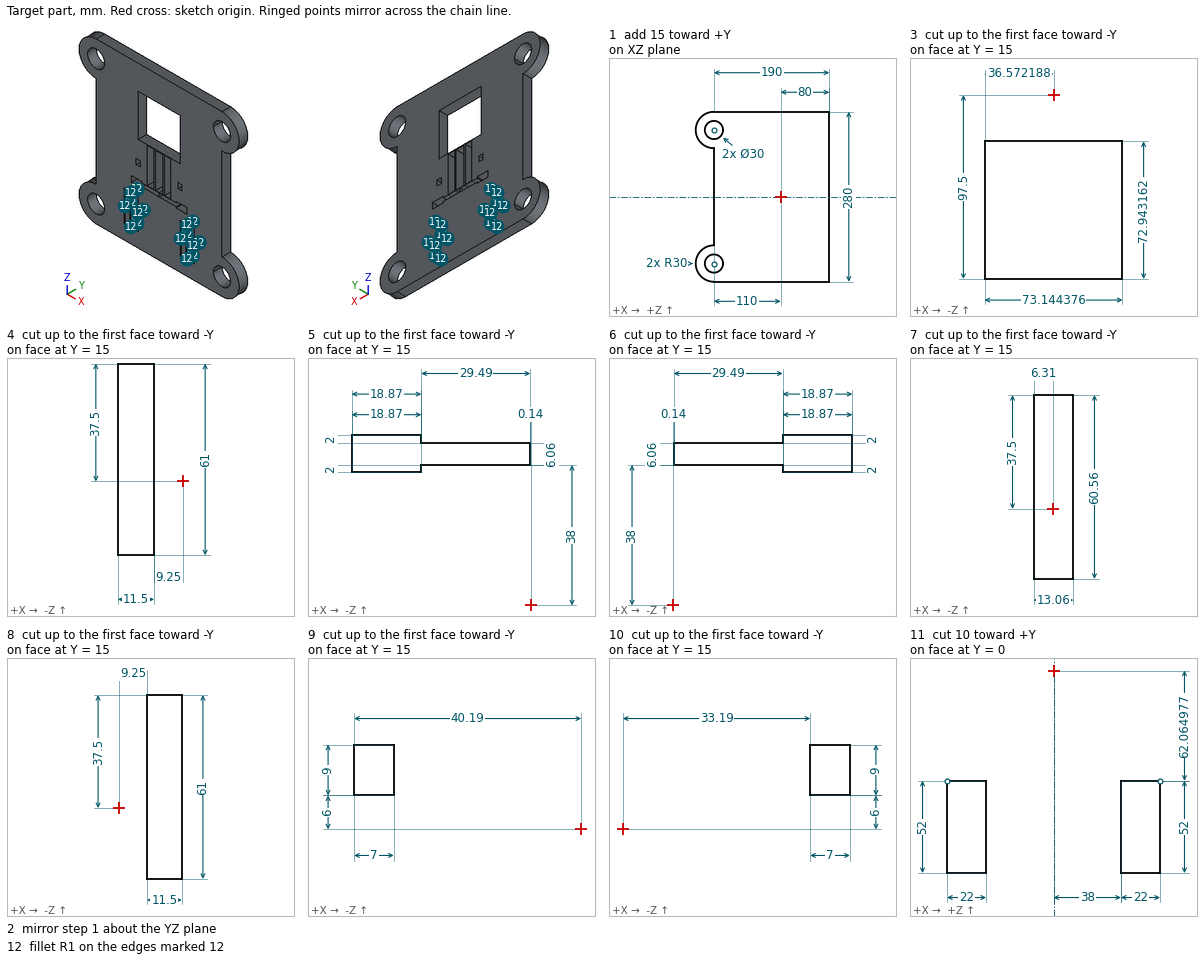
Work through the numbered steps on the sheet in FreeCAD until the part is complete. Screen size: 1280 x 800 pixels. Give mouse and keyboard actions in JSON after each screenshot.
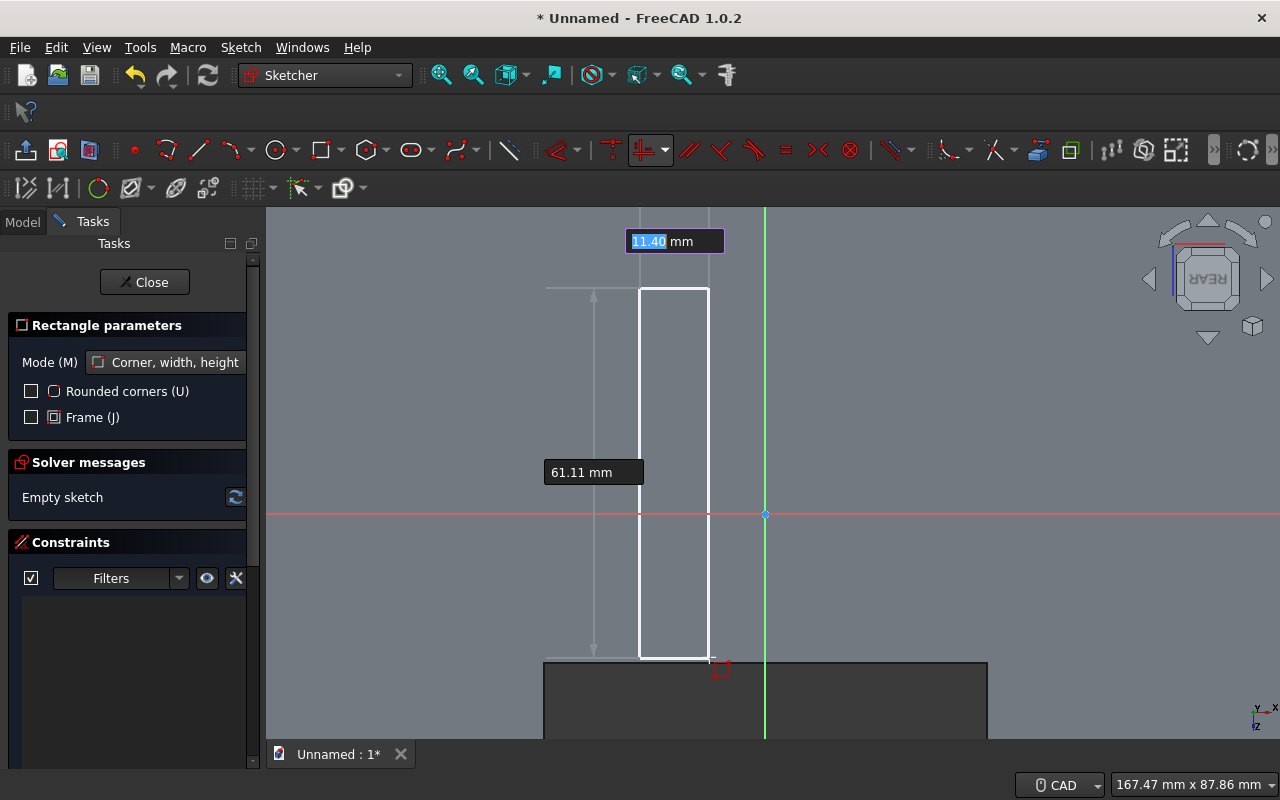
{"action": "type", "text": "11.5"}
{"action": "key", "text": "Tab"}
{"action": "type", "text": "61"}
{"action": "key", "text": "Return"}
{"action": "key", "text": "Escape"}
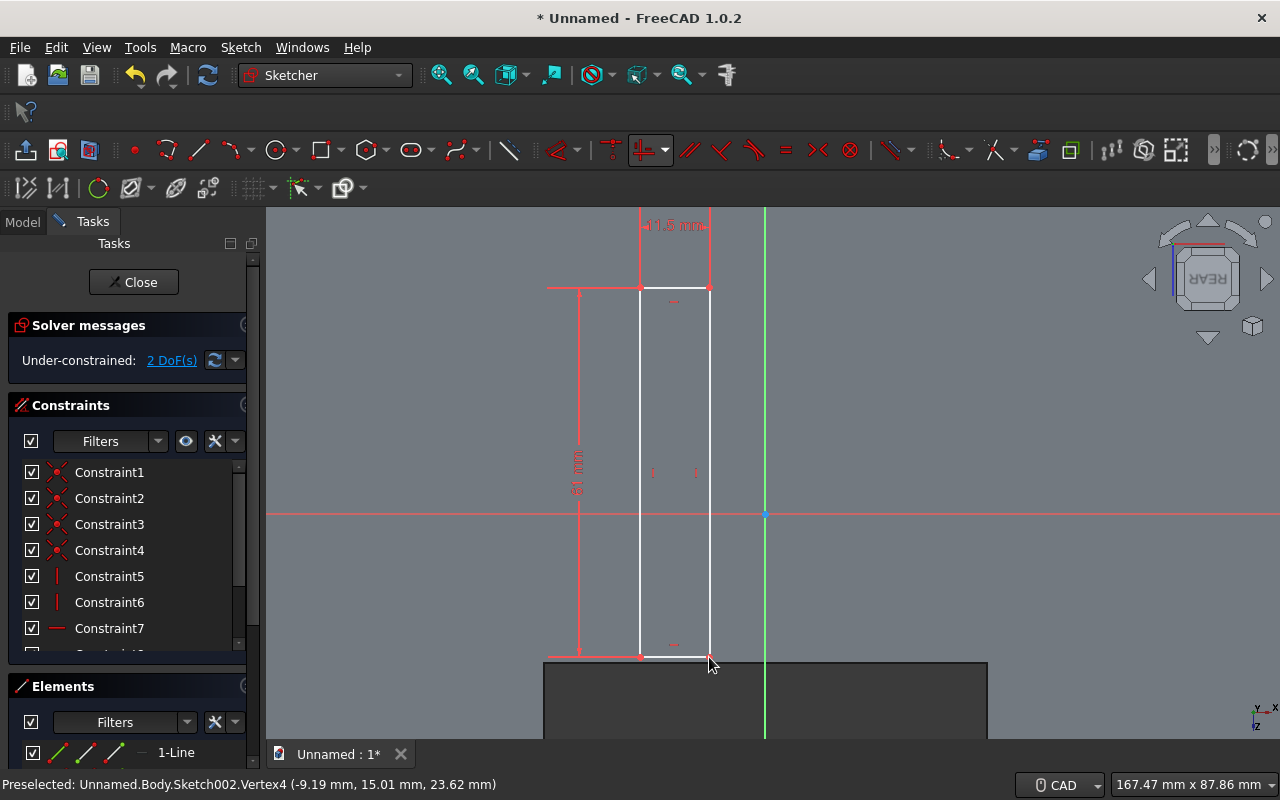
{"action": "left_click", "coordinate": [556, 150]}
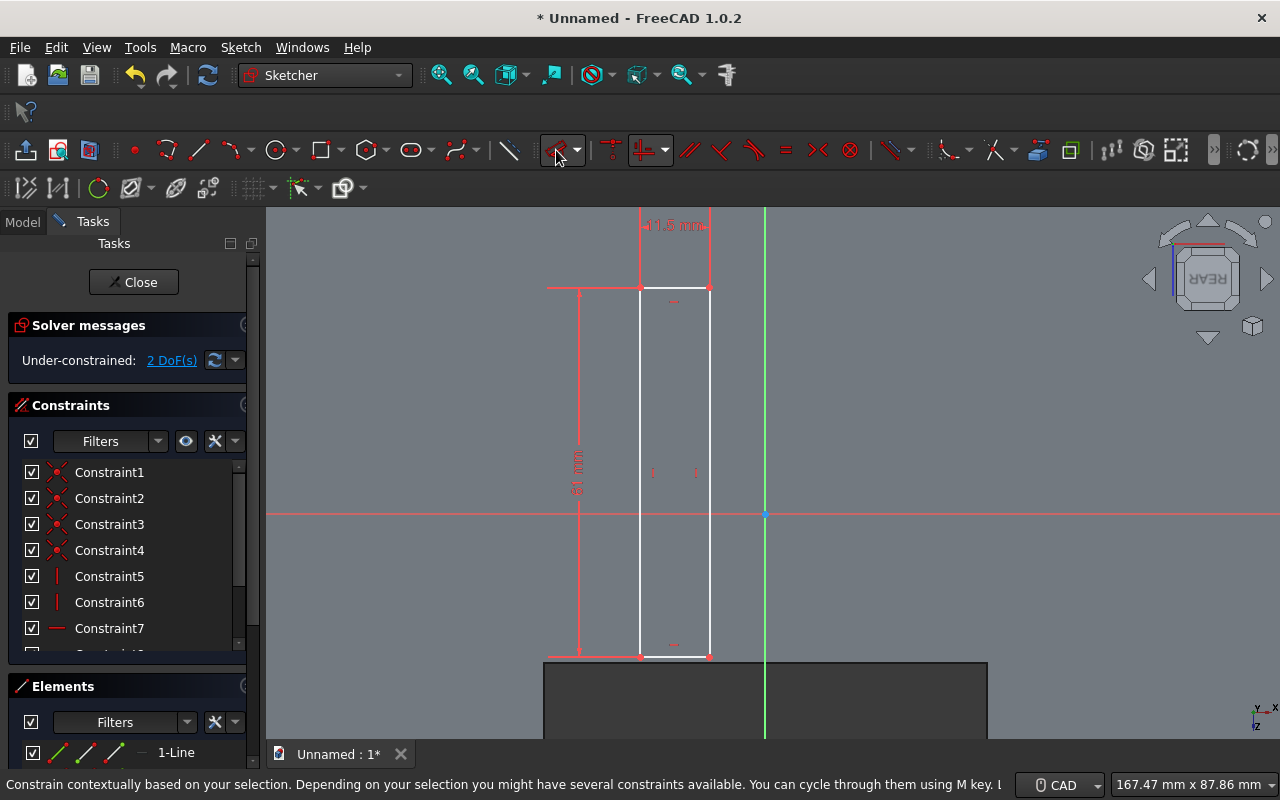
{"action": "left_click", "coordinate": [640, 288]}
{"action": "left_click", "coordinate": [799, 401]}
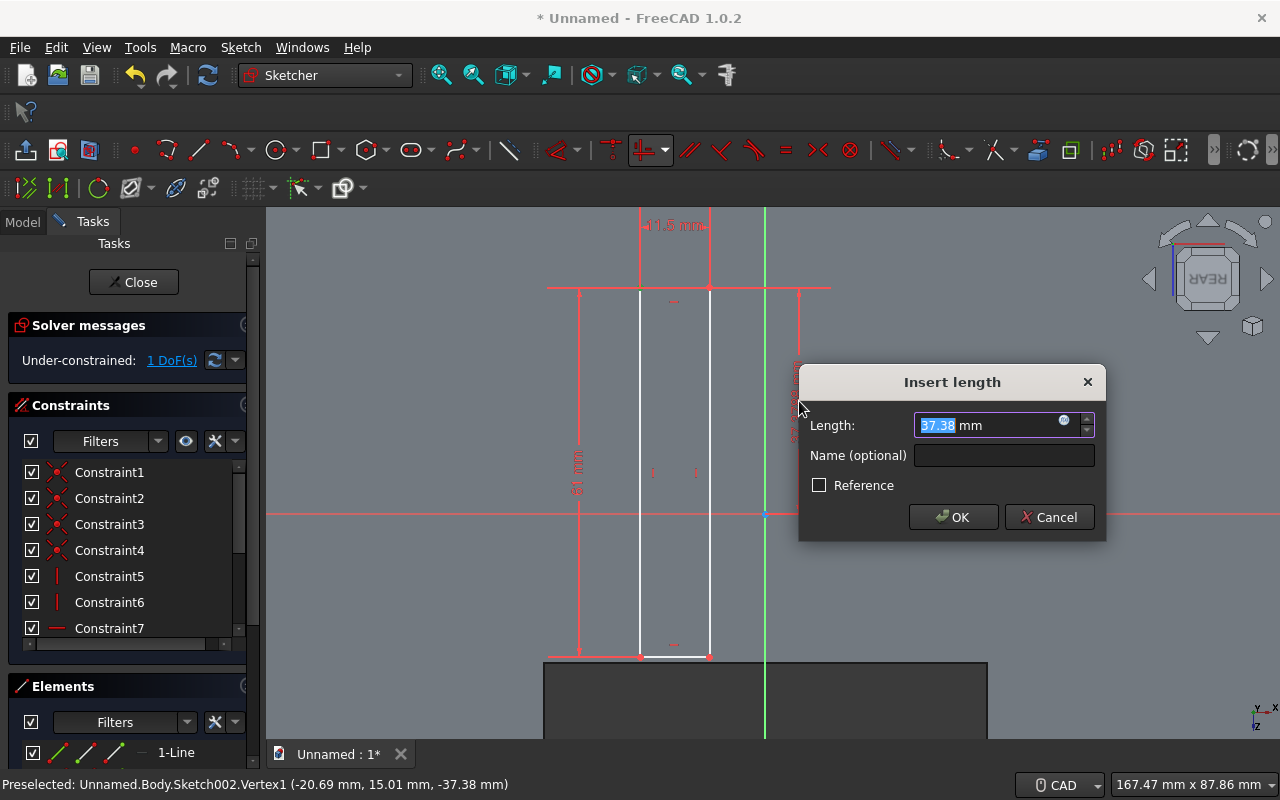
{"action": "type", "text": "37.5"}
{"action": "key", "text": "Return"}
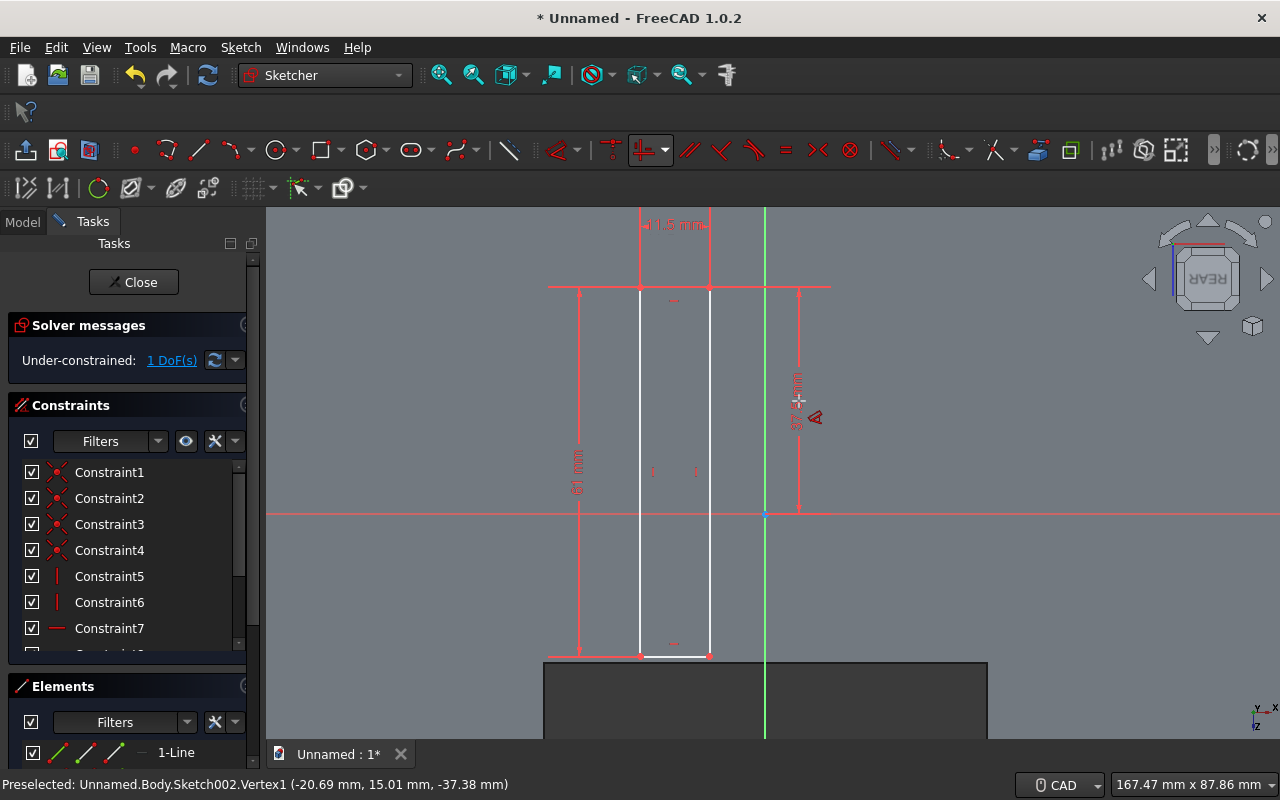
{"action": "left_click", "coordinate": [710, 657]}
{"action": "left_click", "coordinate": [737, 691]}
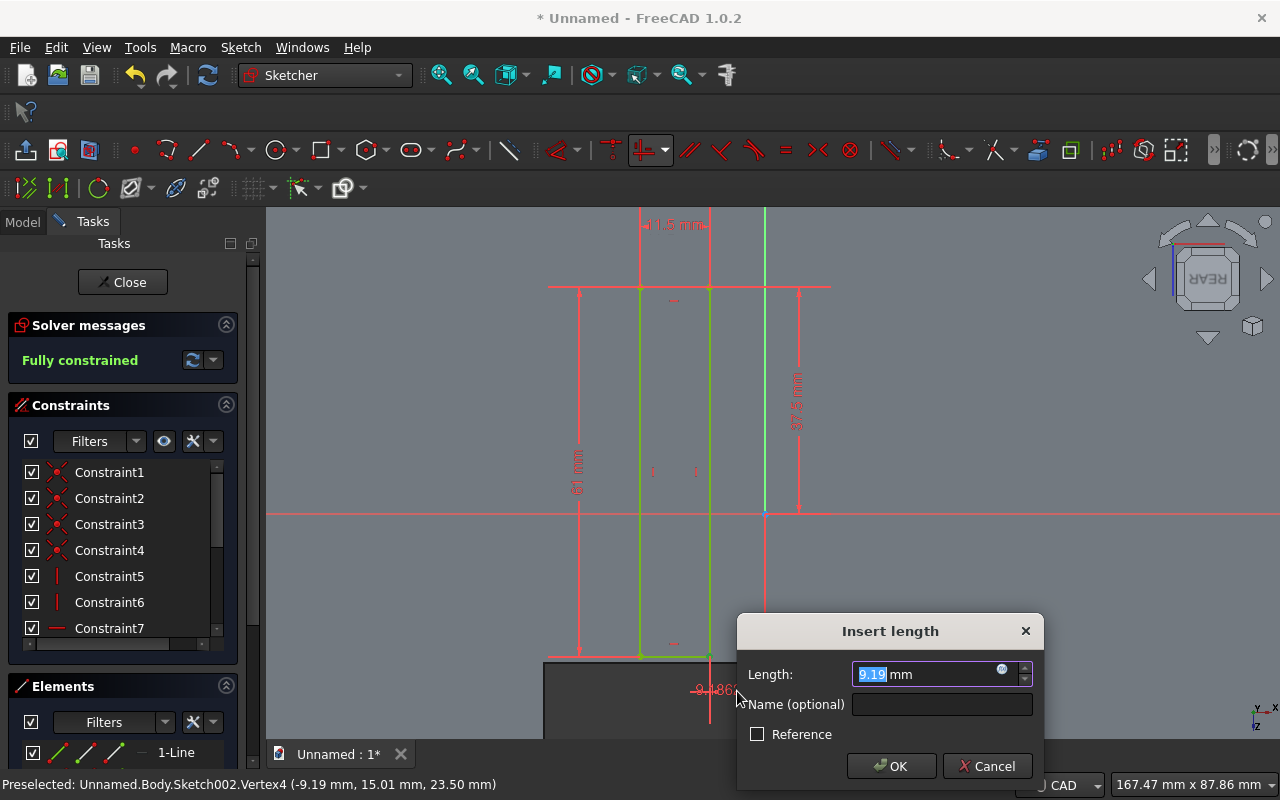
{"action": "type", "text": "9.25"}
{"action": "key", "text": "Return"}
{"action": "key", "text": "Escape"}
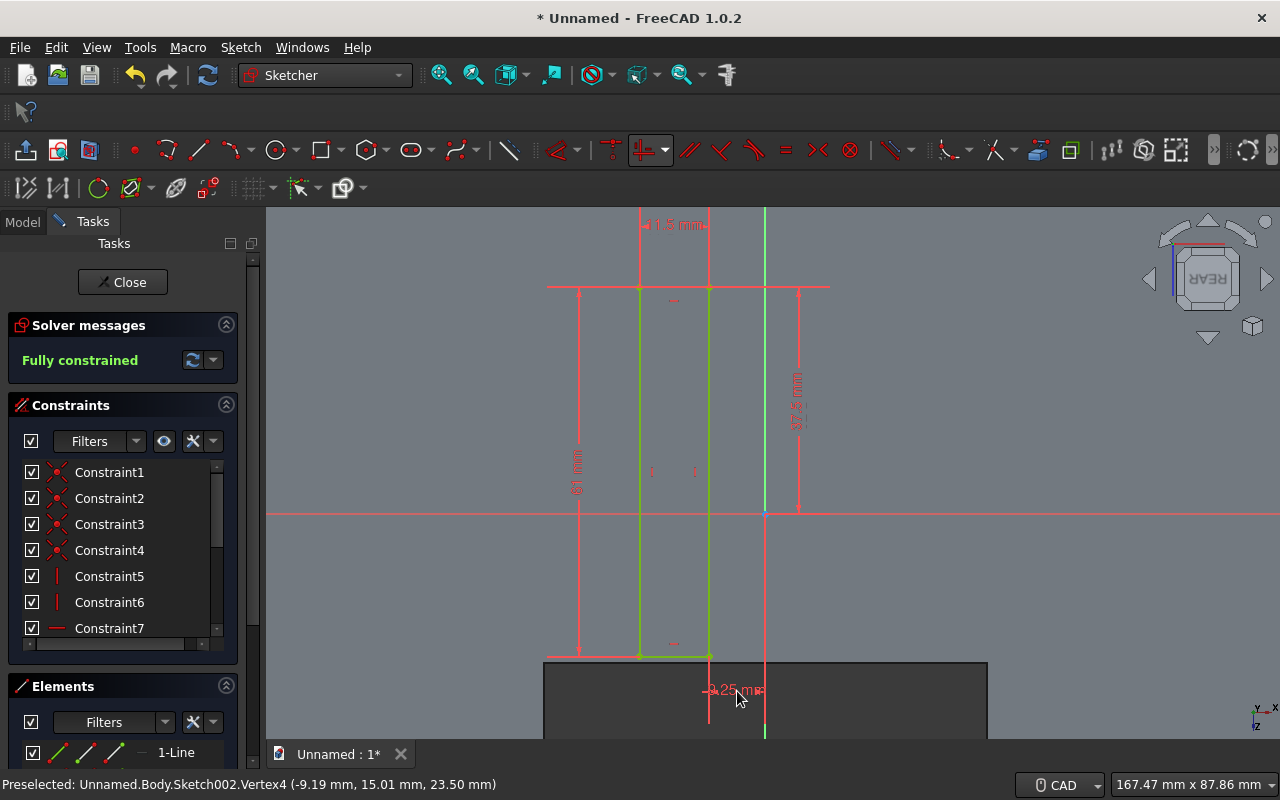
{"action": "left_click", "coordinate": [123, 282]}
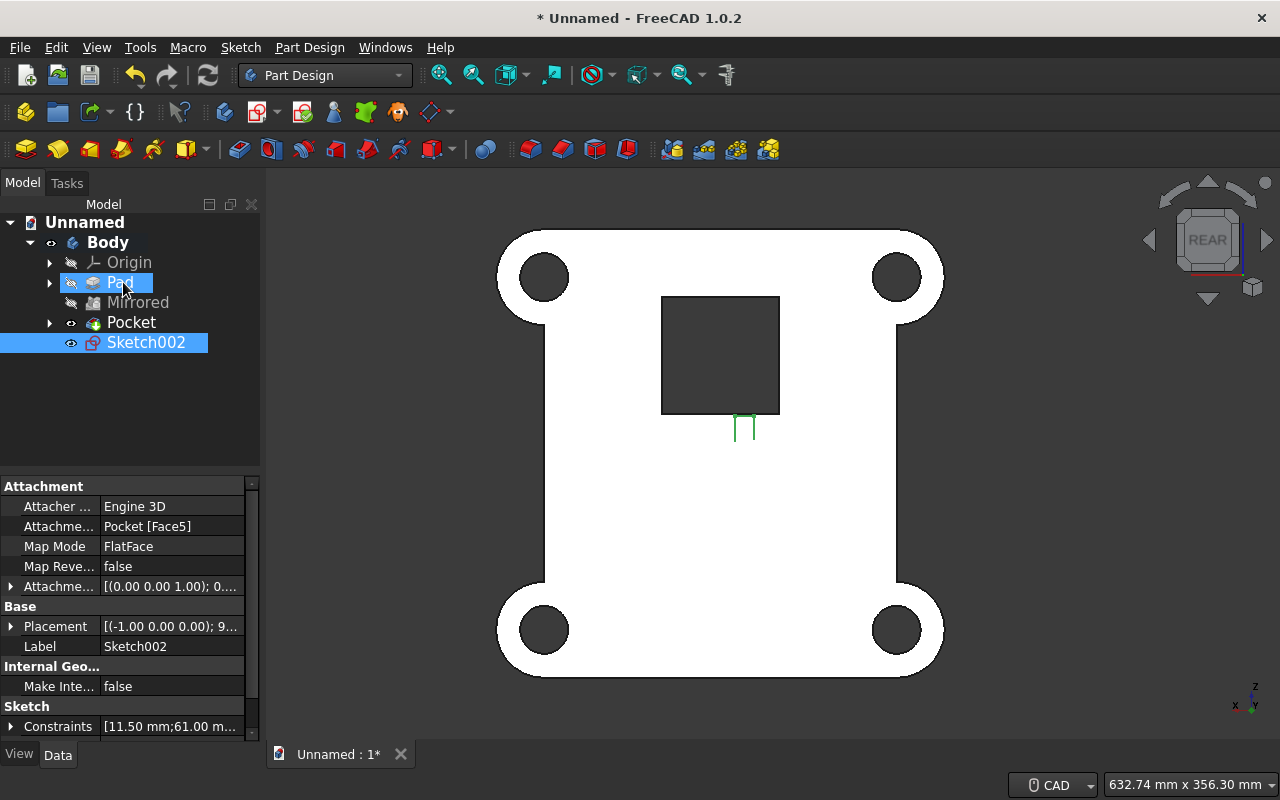
{"action": "left_click", "coordinate": [240, 150]}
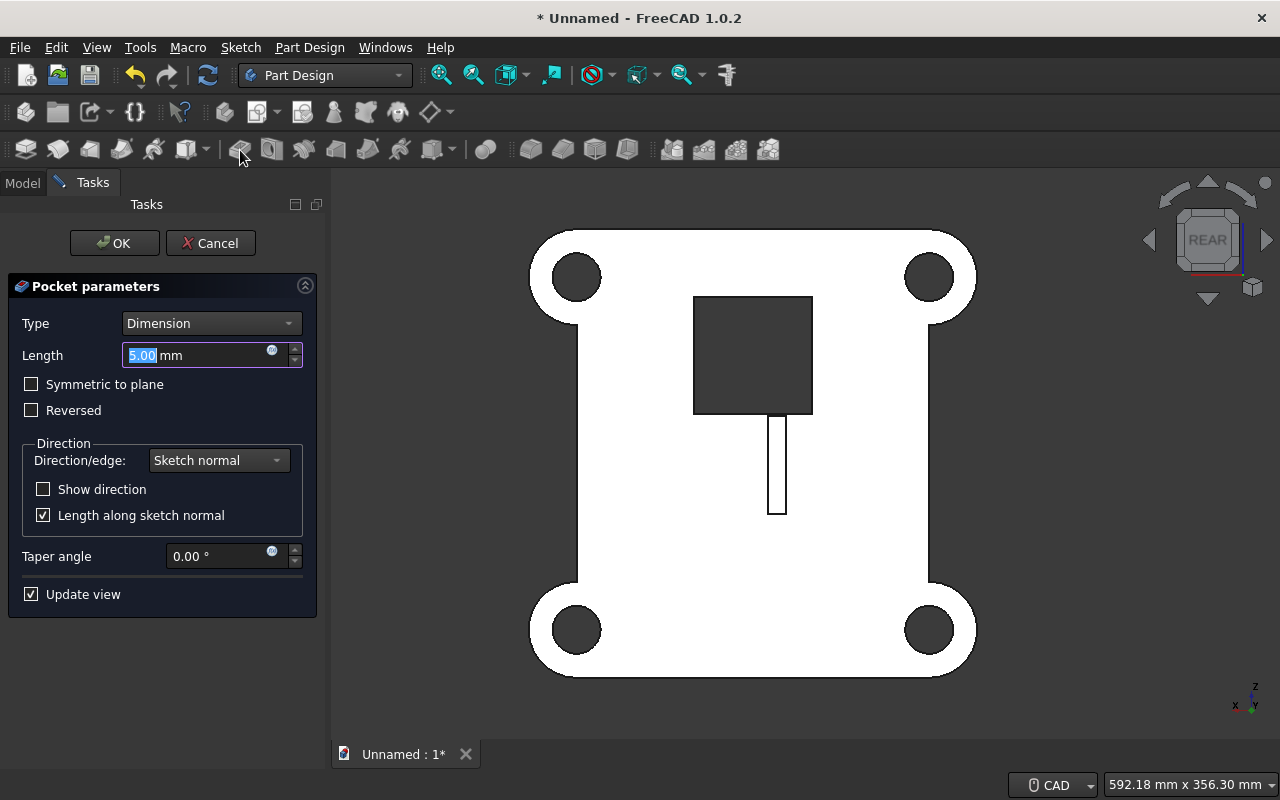
{"action": "left_click", "coordinate": [212, 324]}